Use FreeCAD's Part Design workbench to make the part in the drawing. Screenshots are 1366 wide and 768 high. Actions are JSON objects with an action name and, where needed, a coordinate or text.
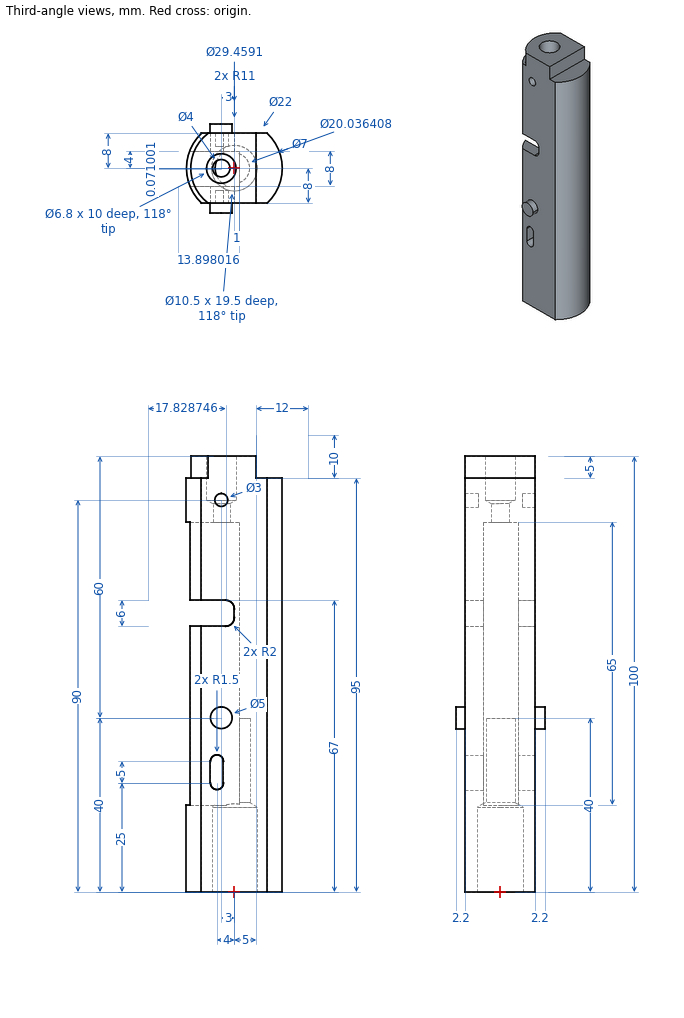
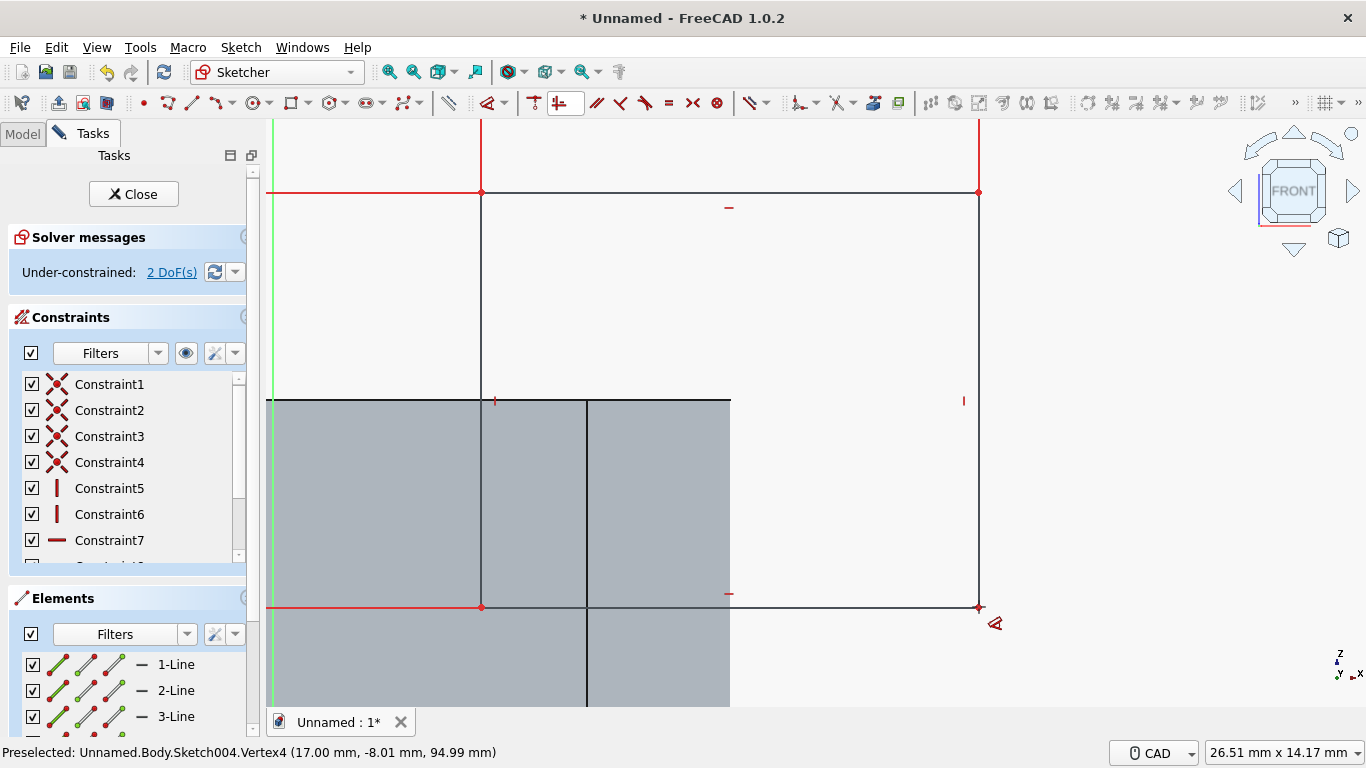
{"action": "left_click", "coordinate": [481, 193]}
{"action": "left_click", "coordinate": [387, 159]}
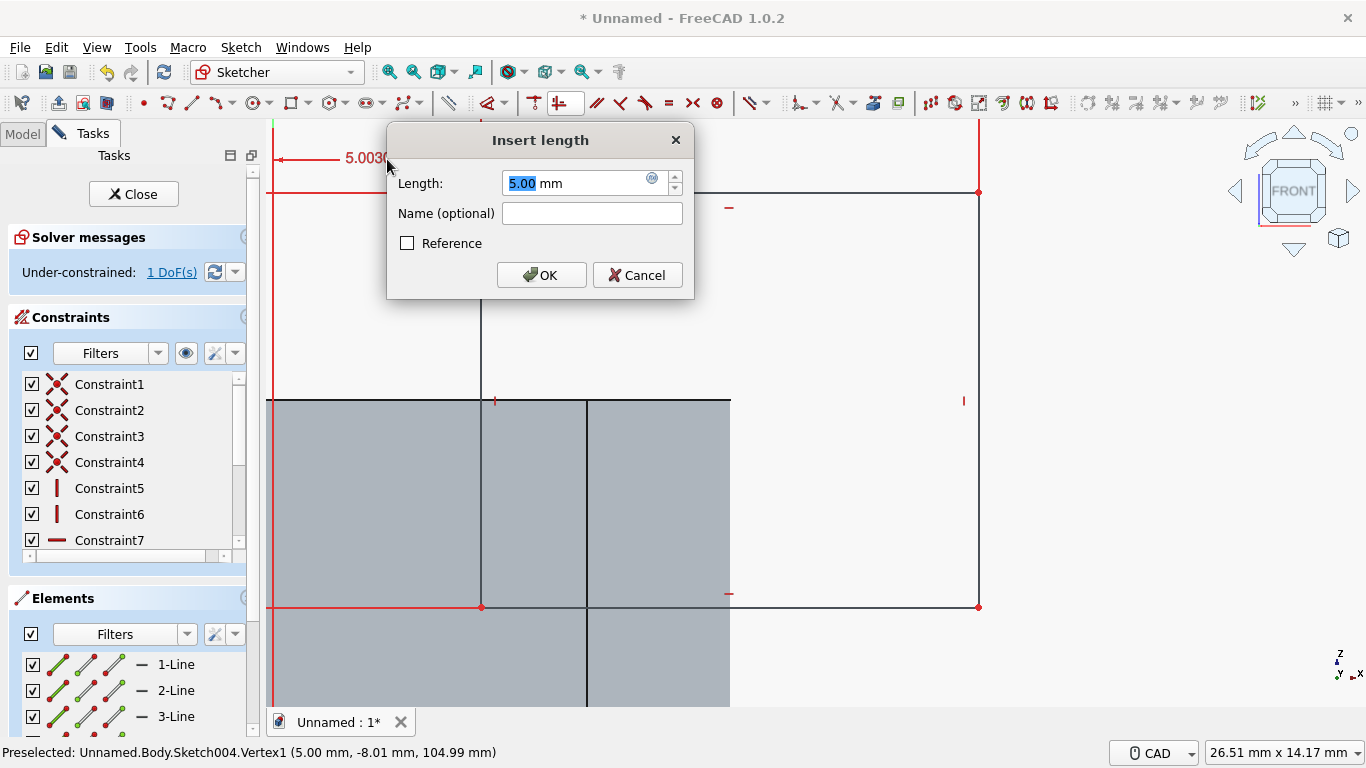
{"action": "type", "text": "5"}
{"action": "key", "text": "Return"}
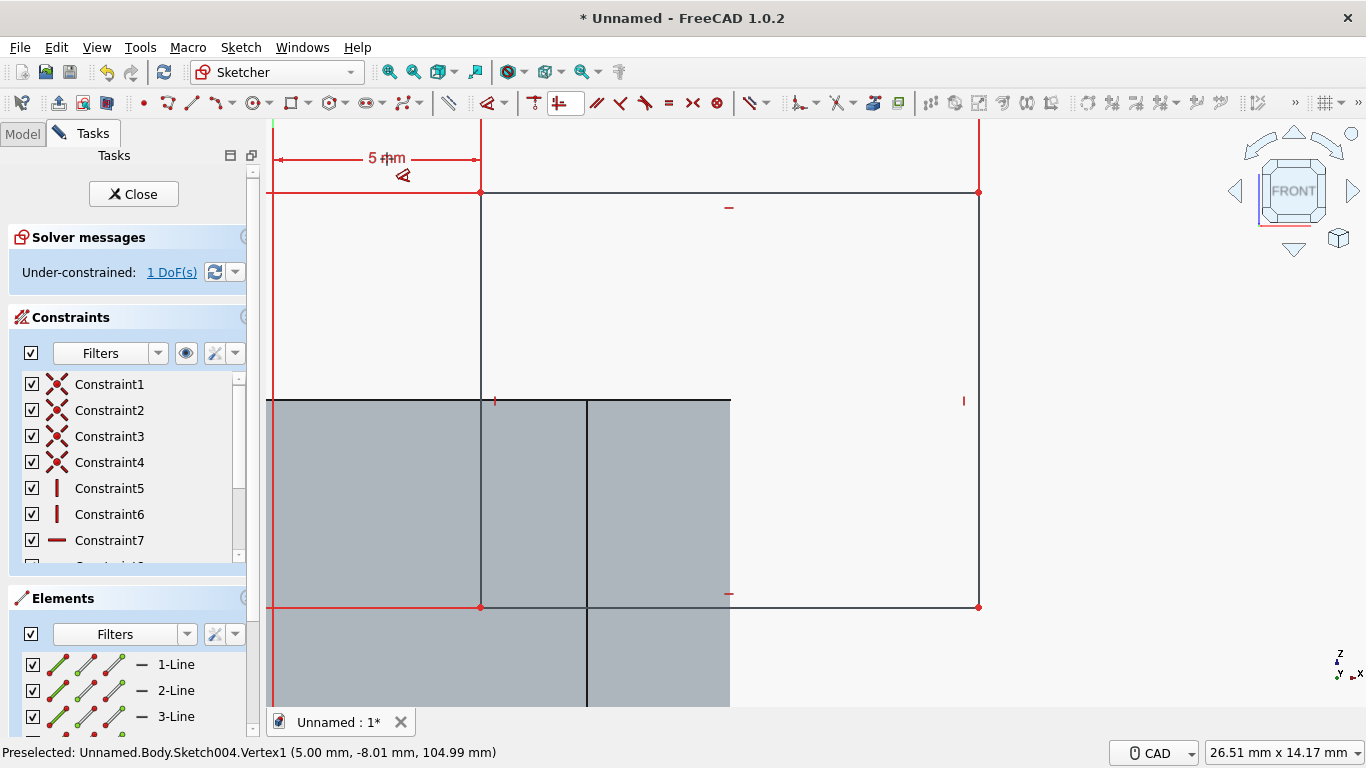
{"action": "left_click", "coordinate": [481, 608]}
{"action": "left_click", "coordinate": [515, 643]}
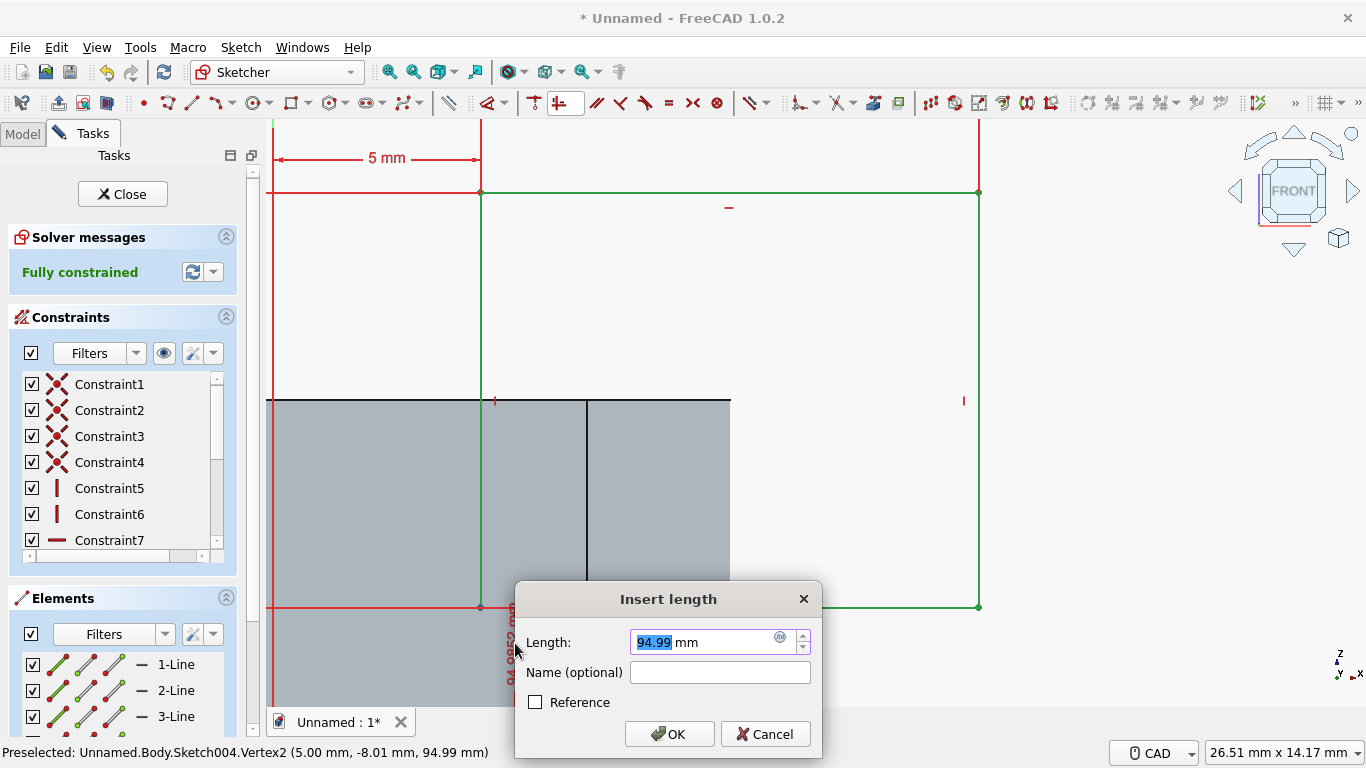
{"action": "type", "text": "95"}
{"action": "key", "text": "Return"}
{"action": "key", "text": "Escape"}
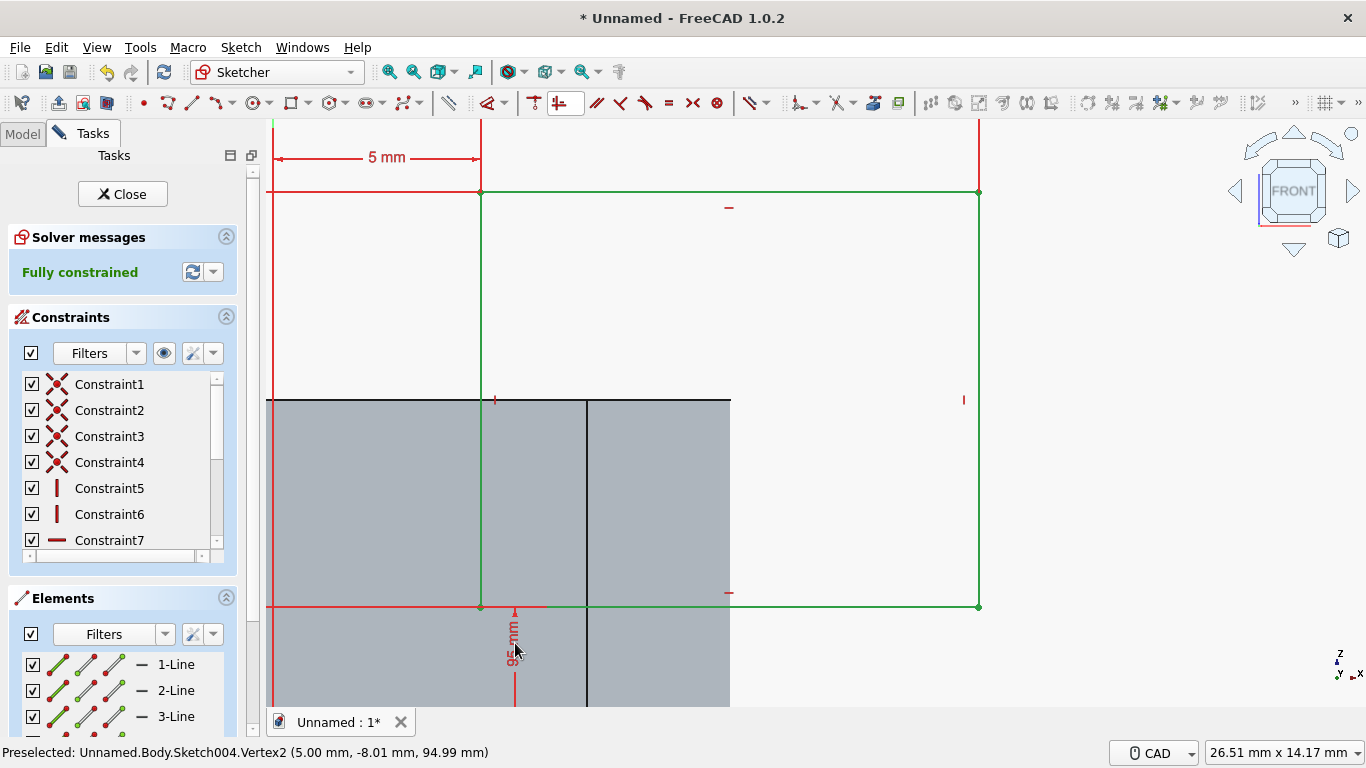
{"action": "left_click", "coordinate": [123, 194]}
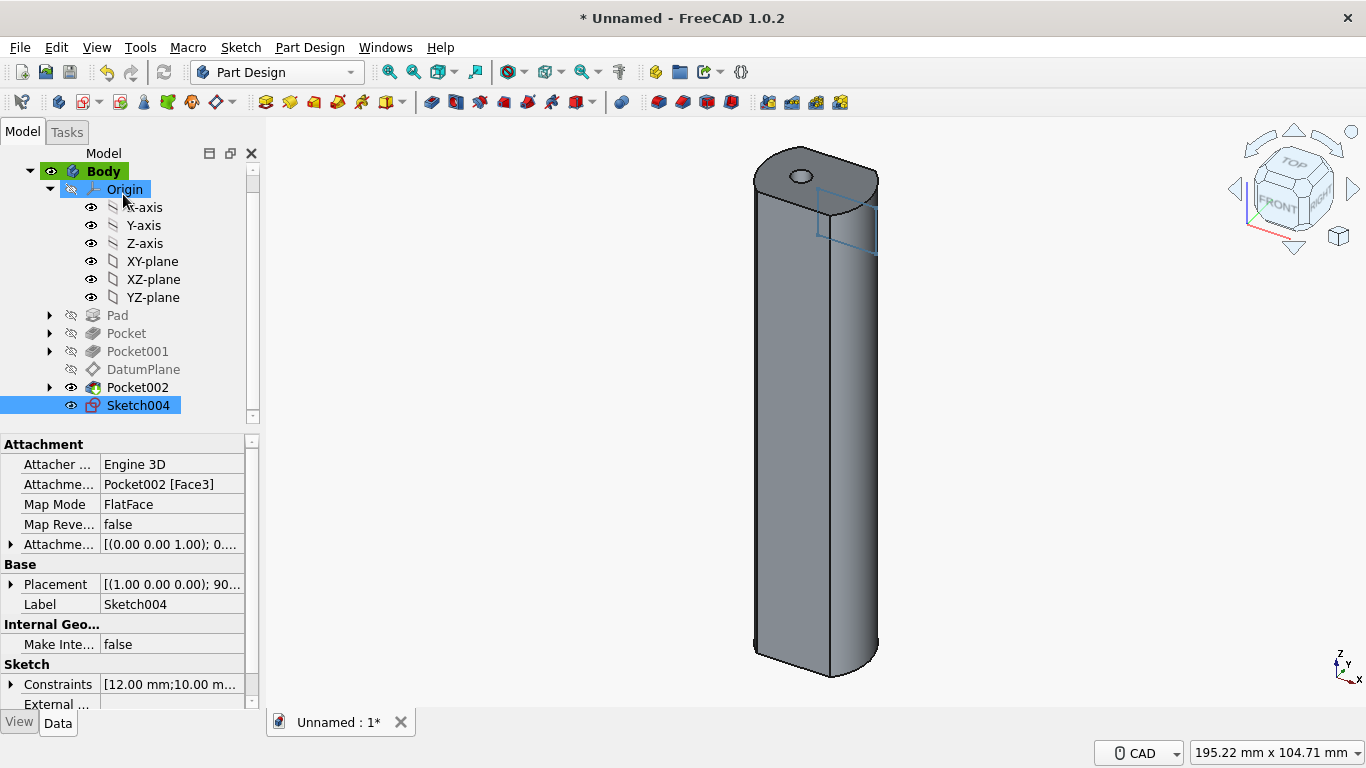
{"action": "left_click", "coordinate": [432, 102]}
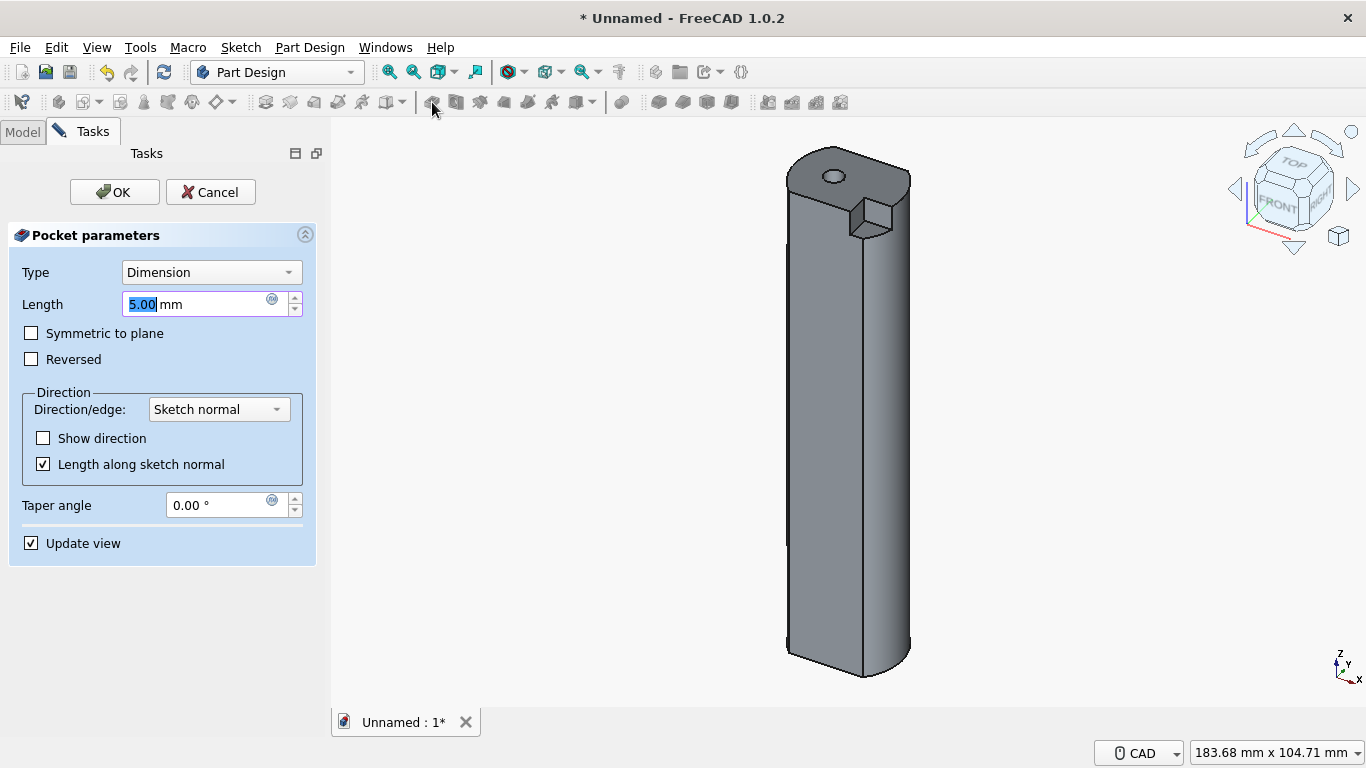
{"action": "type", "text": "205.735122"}
{"action": "key", "text": "Tab"}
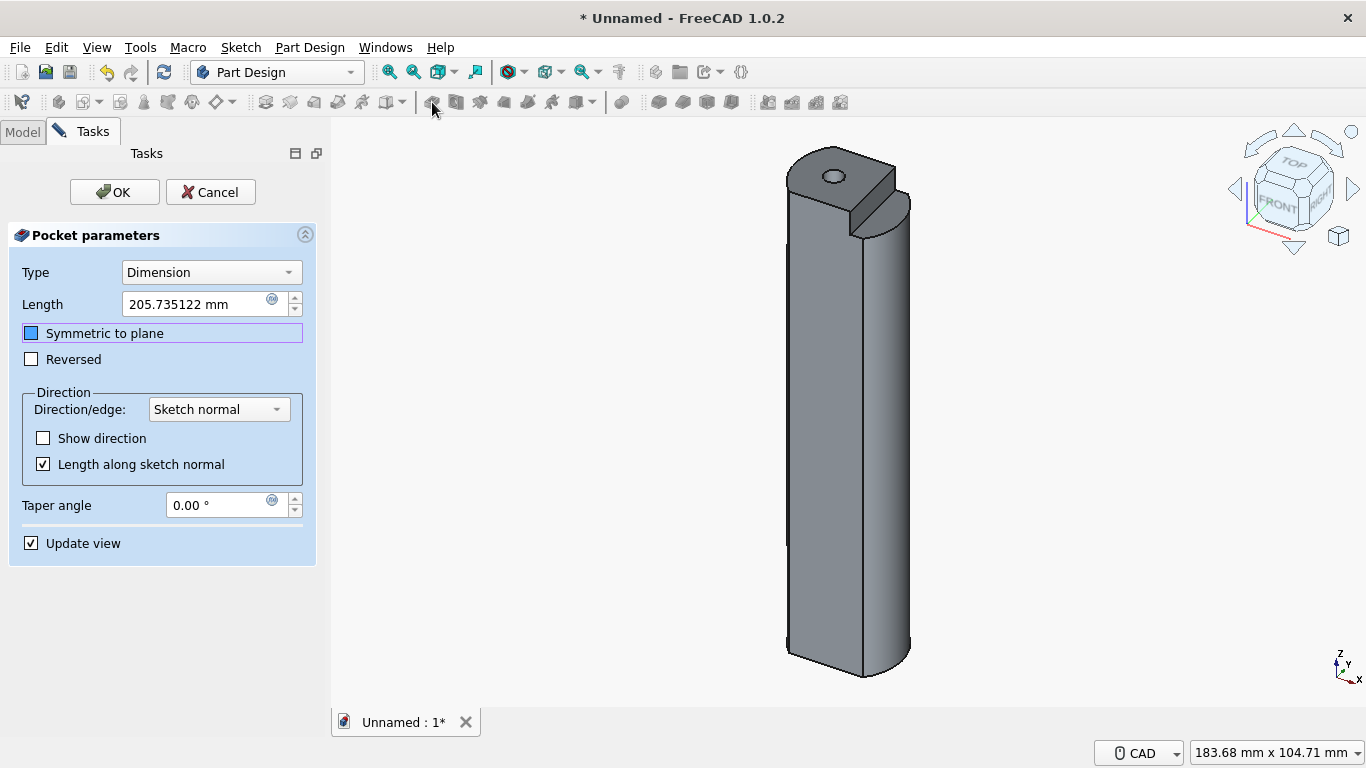
{"action": "left_click", "coordinate": [30, 333]}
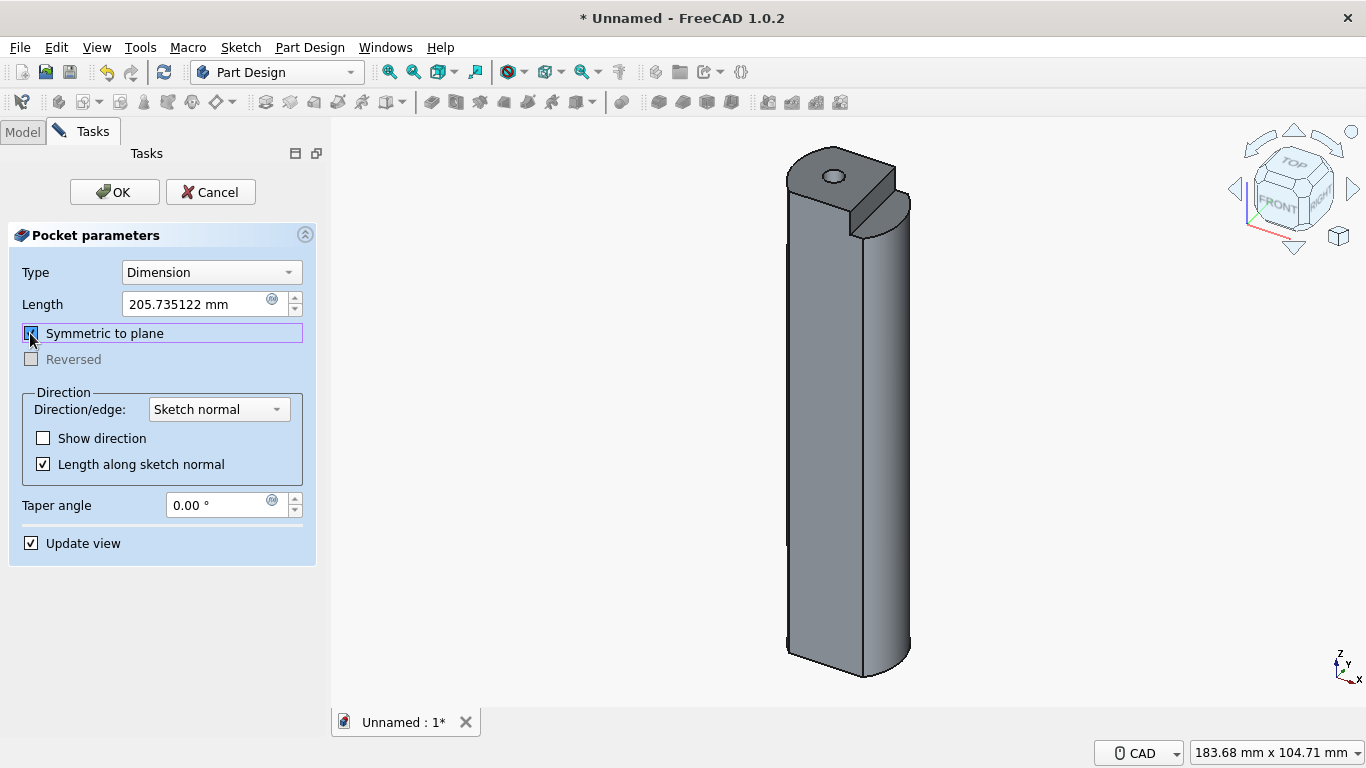
{"action": "left_click", "coordinate": [115, 192]}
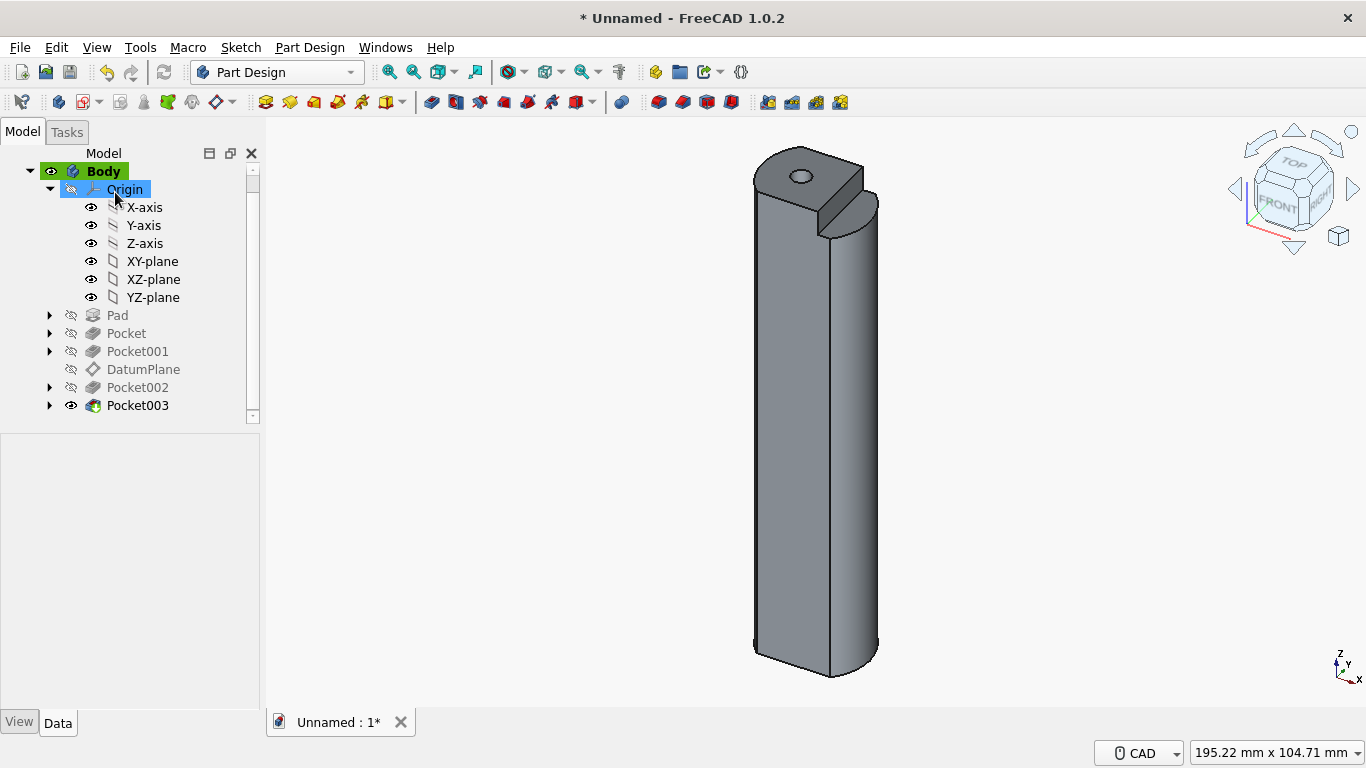
{"action": "left_click", "coordinate": [837, 170]}